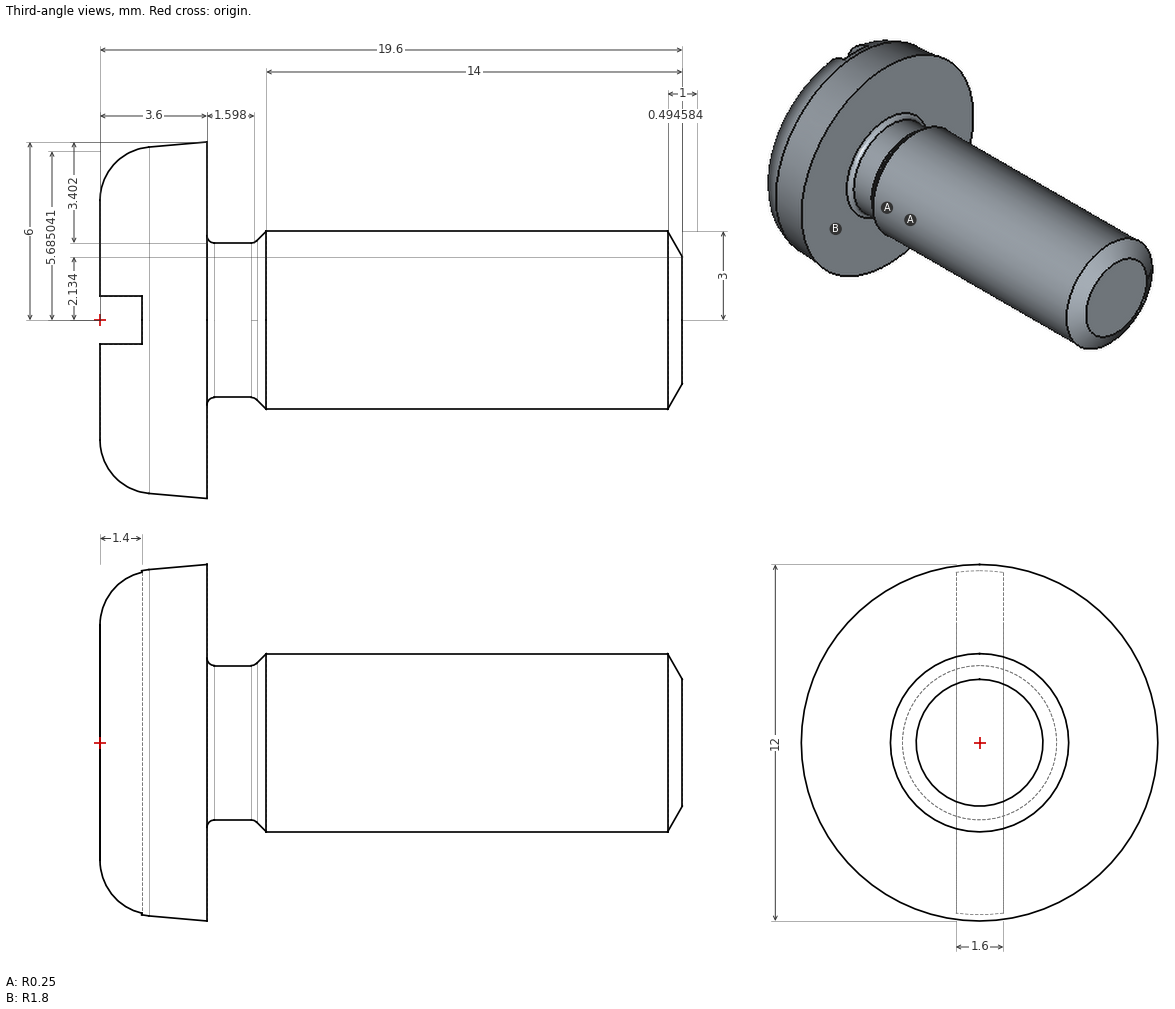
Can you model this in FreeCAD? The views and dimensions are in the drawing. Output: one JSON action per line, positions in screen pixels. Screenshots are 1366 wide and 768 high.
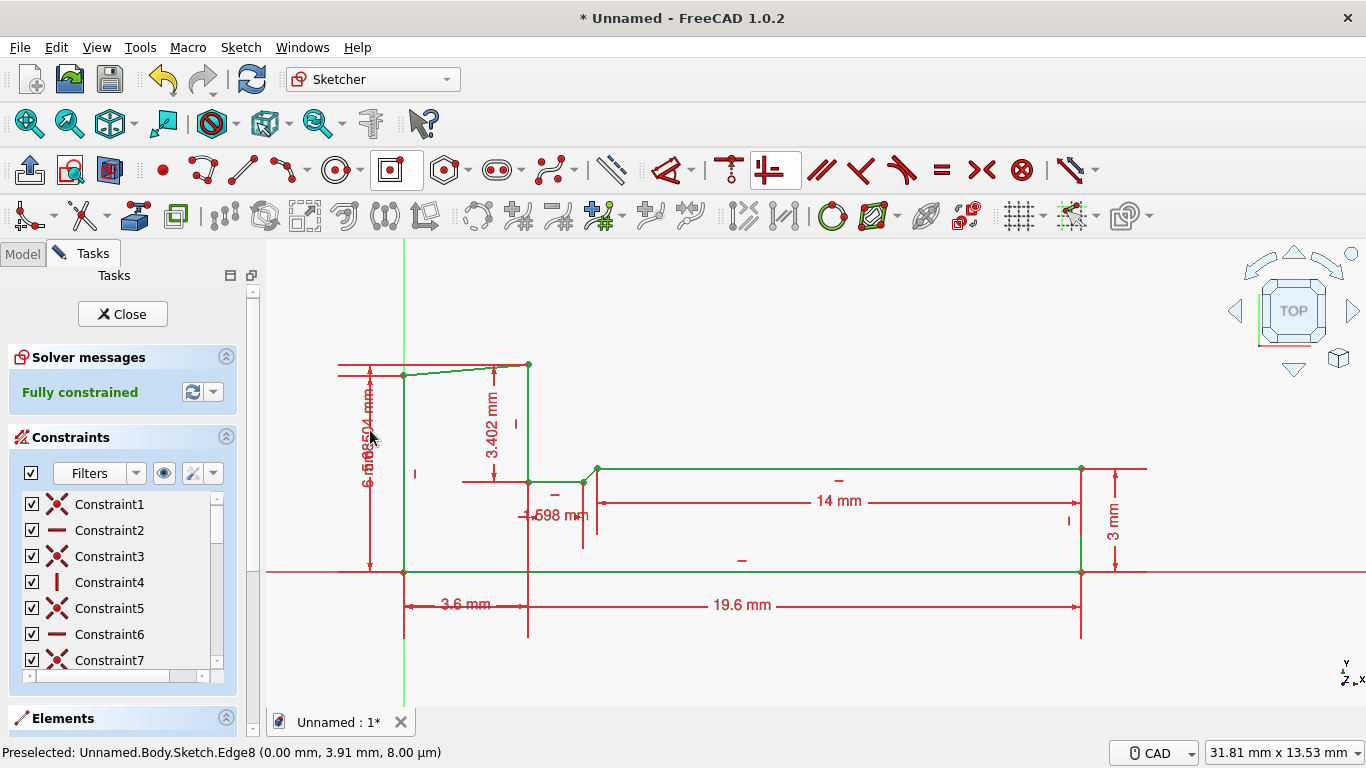
{"action": "left_click", "coordinate": [123, 314]}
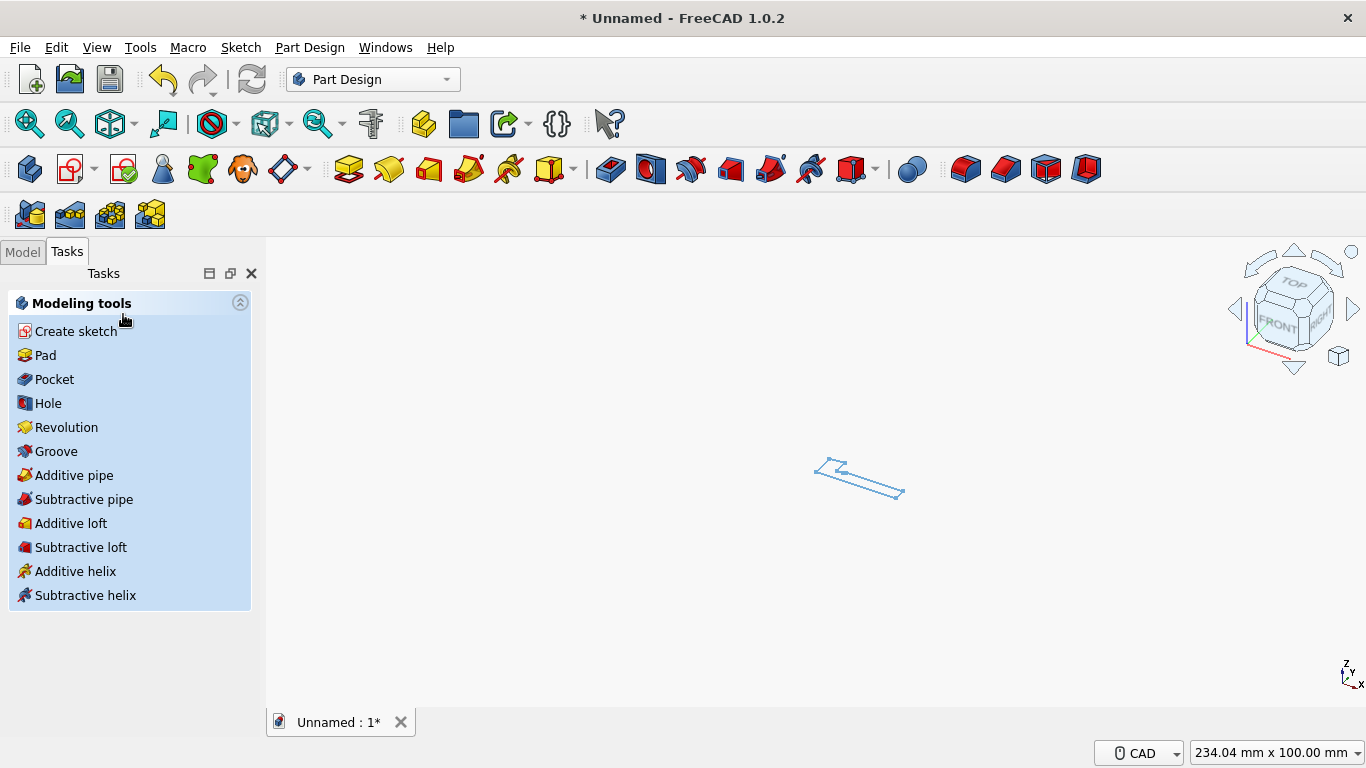
{"action": "left_click", "coordinate": [390, 170]}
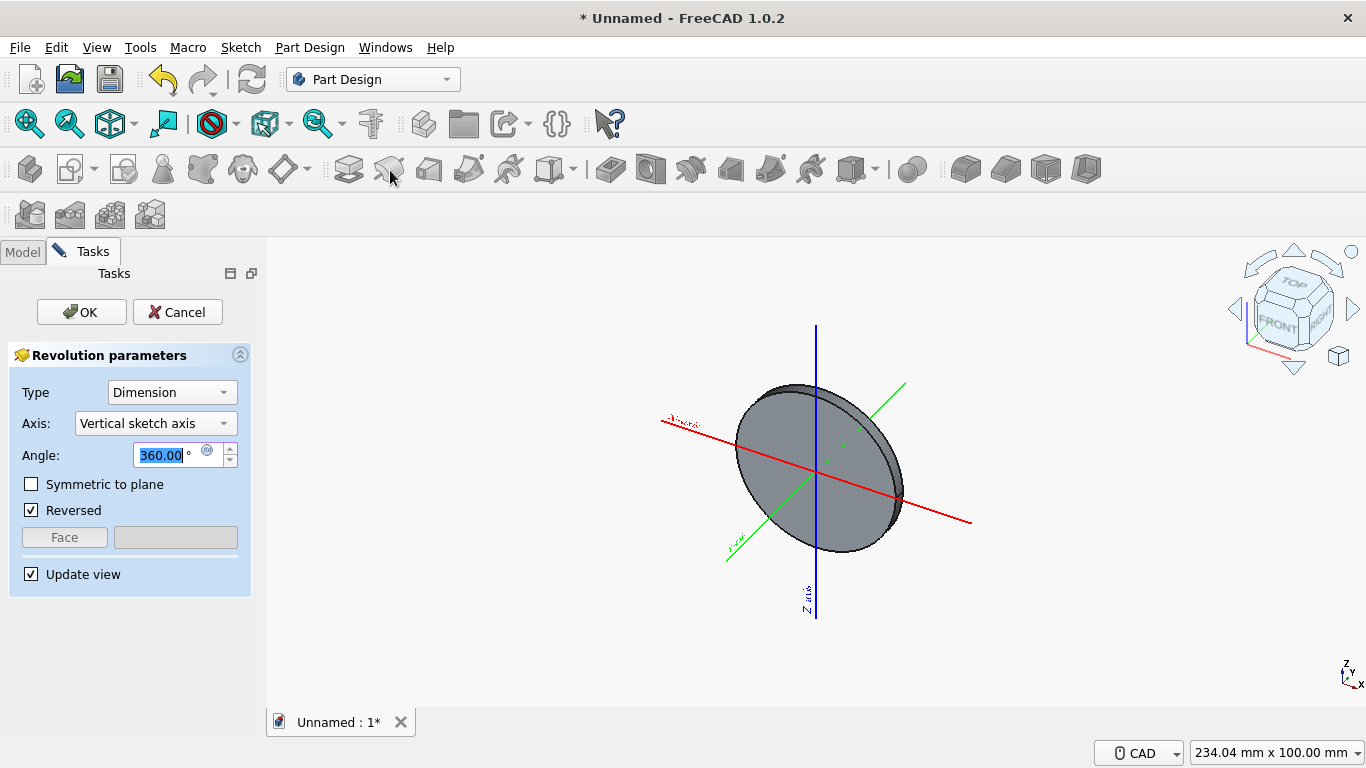
{"action": "left_click", "coordinate": [156, 424]}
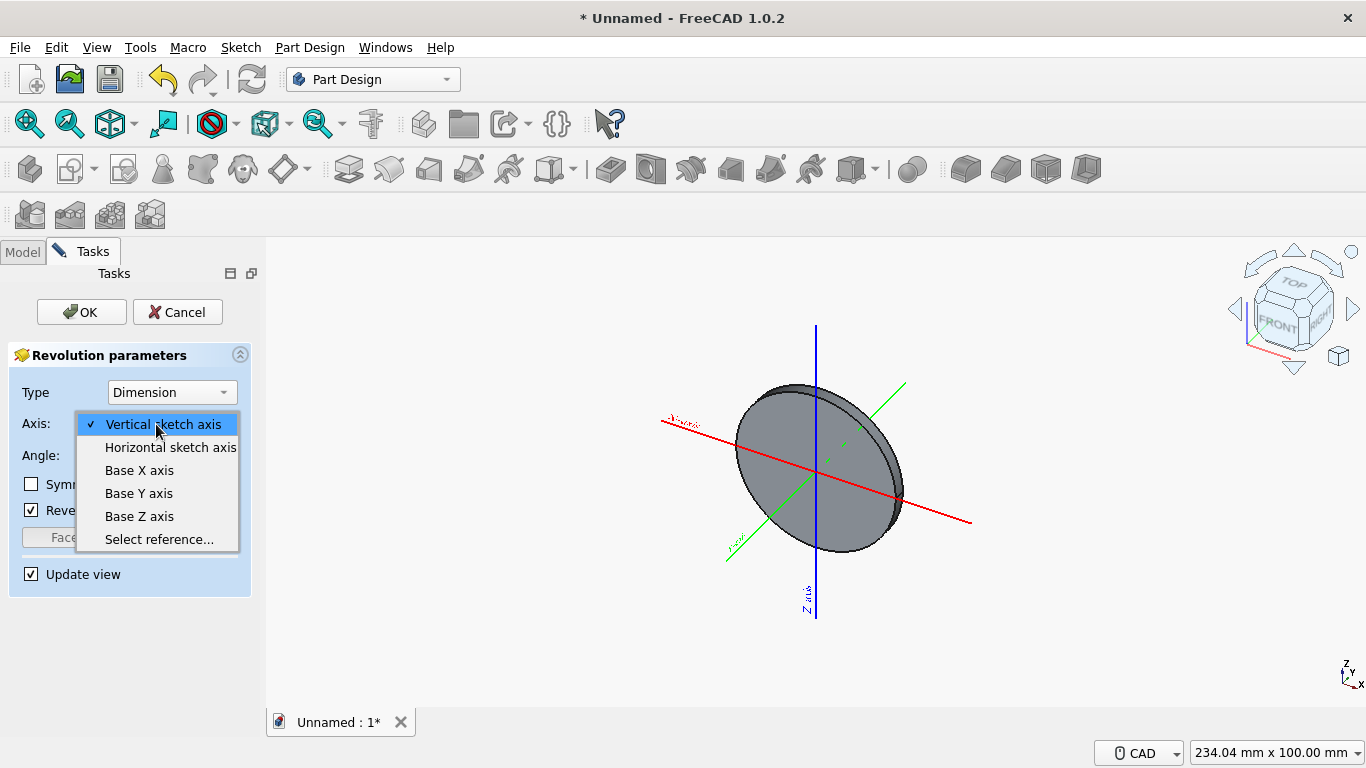
{"action": "left_click", "coordinate": [156, 448]}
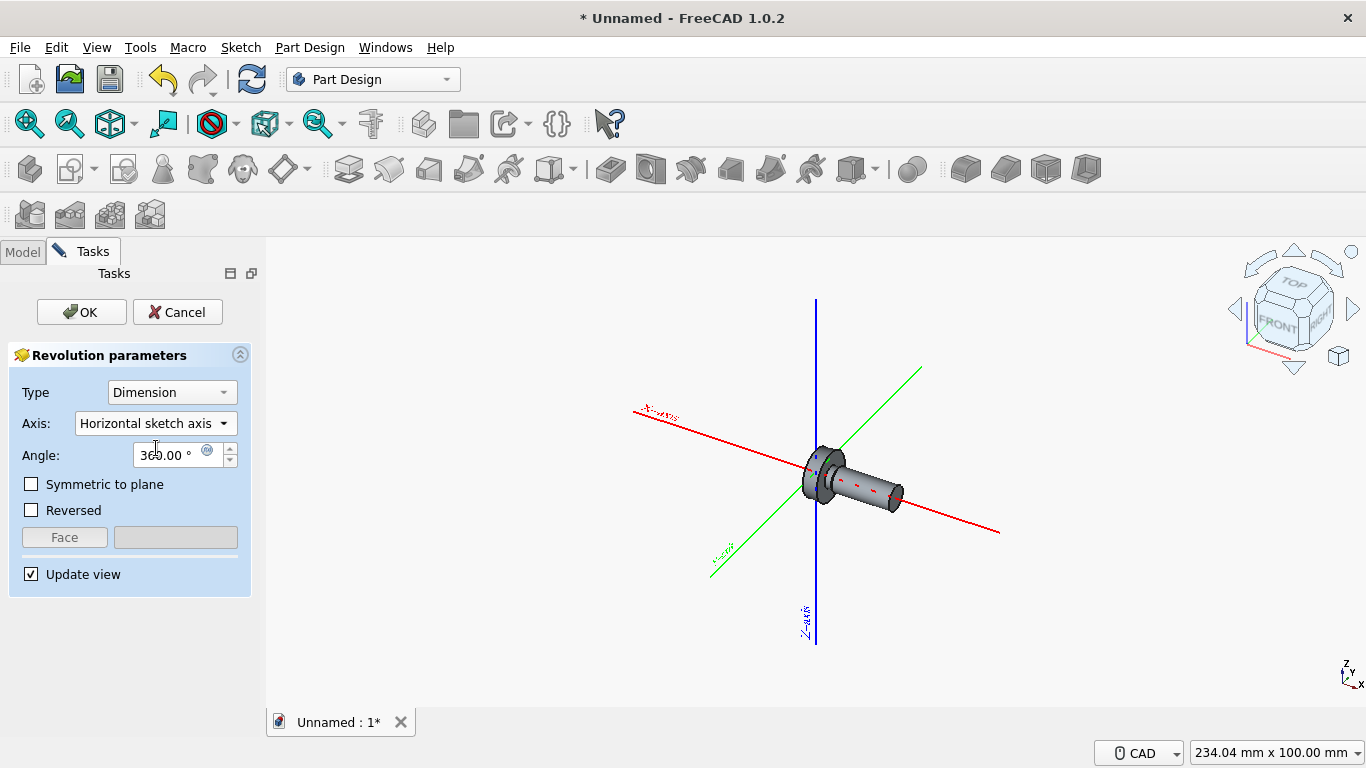
{"action": "left_click", "coordinate": [82, 312]}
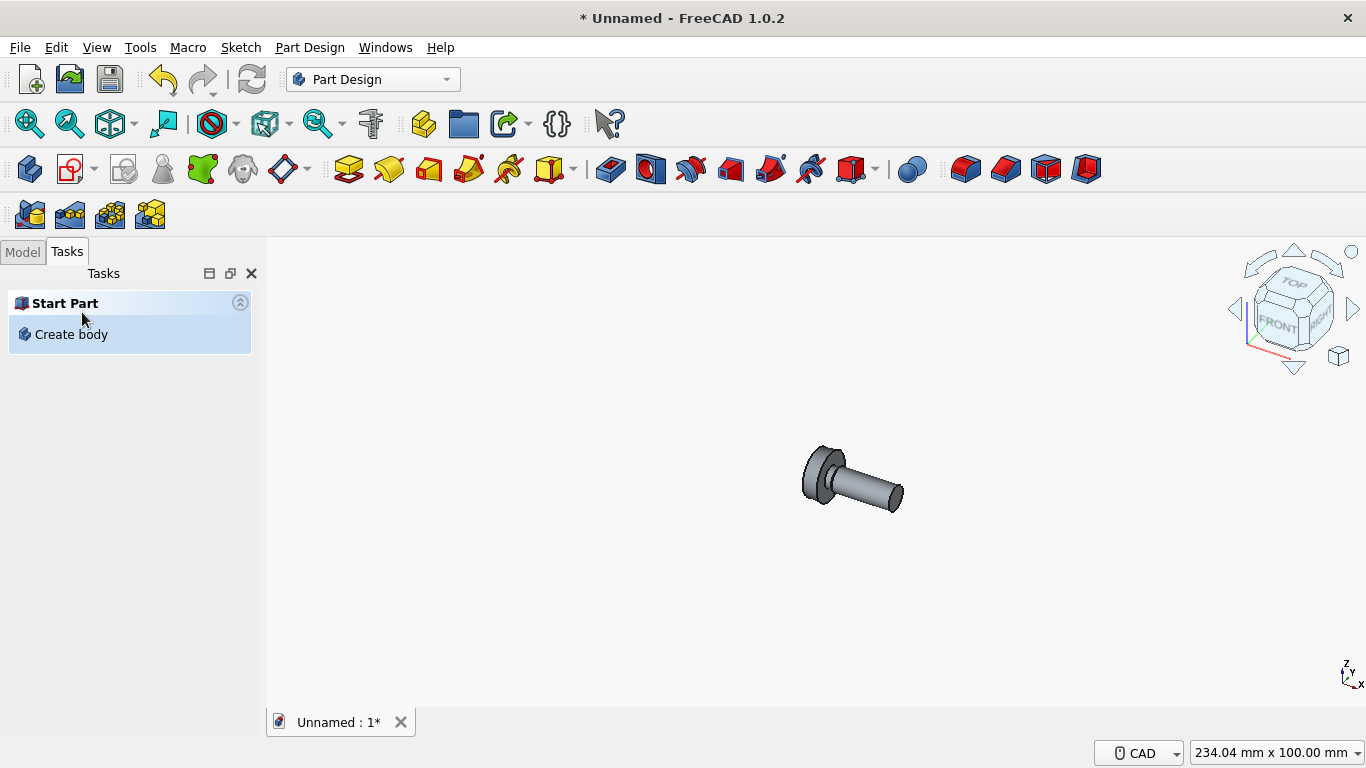
{"action": "left_click", "coordinate": [30, 124]}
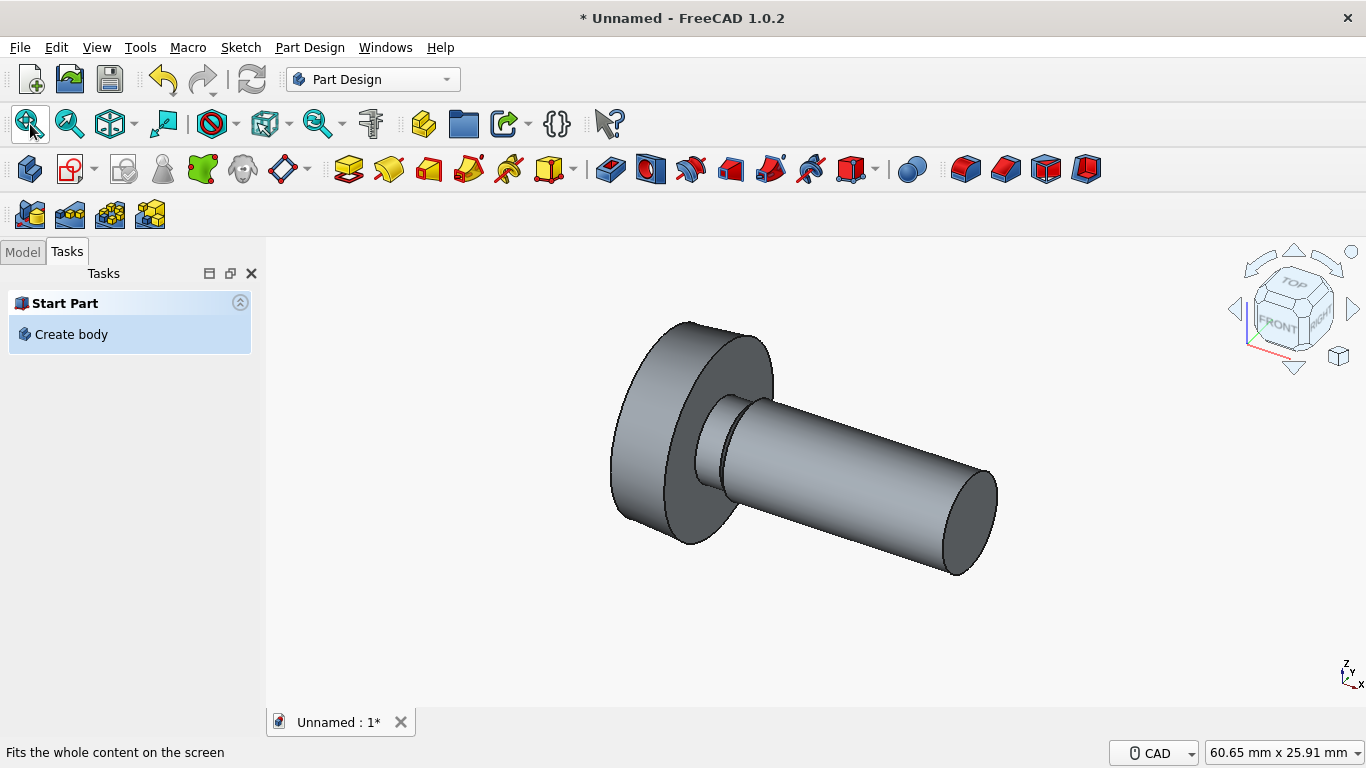
{"action": "key", "text": "0"}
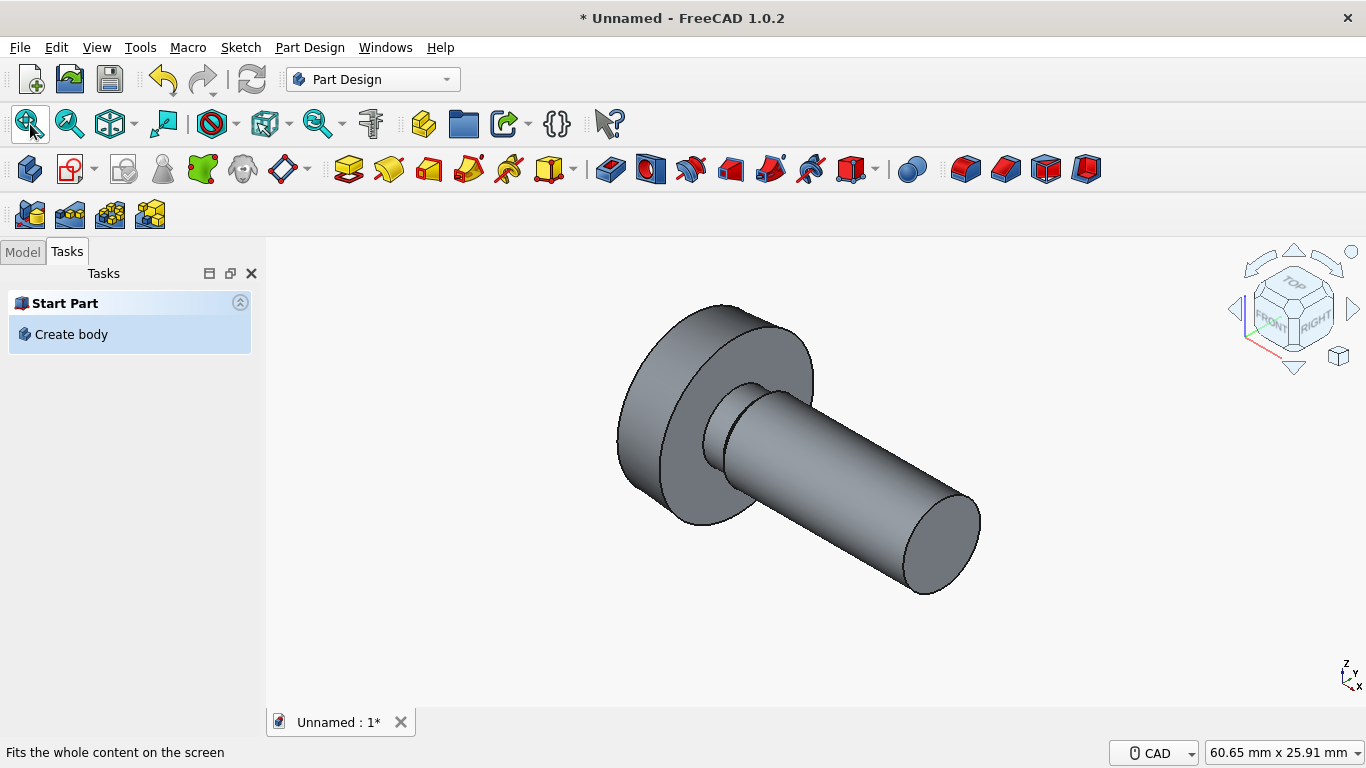
{"action": "key", "text": "2"}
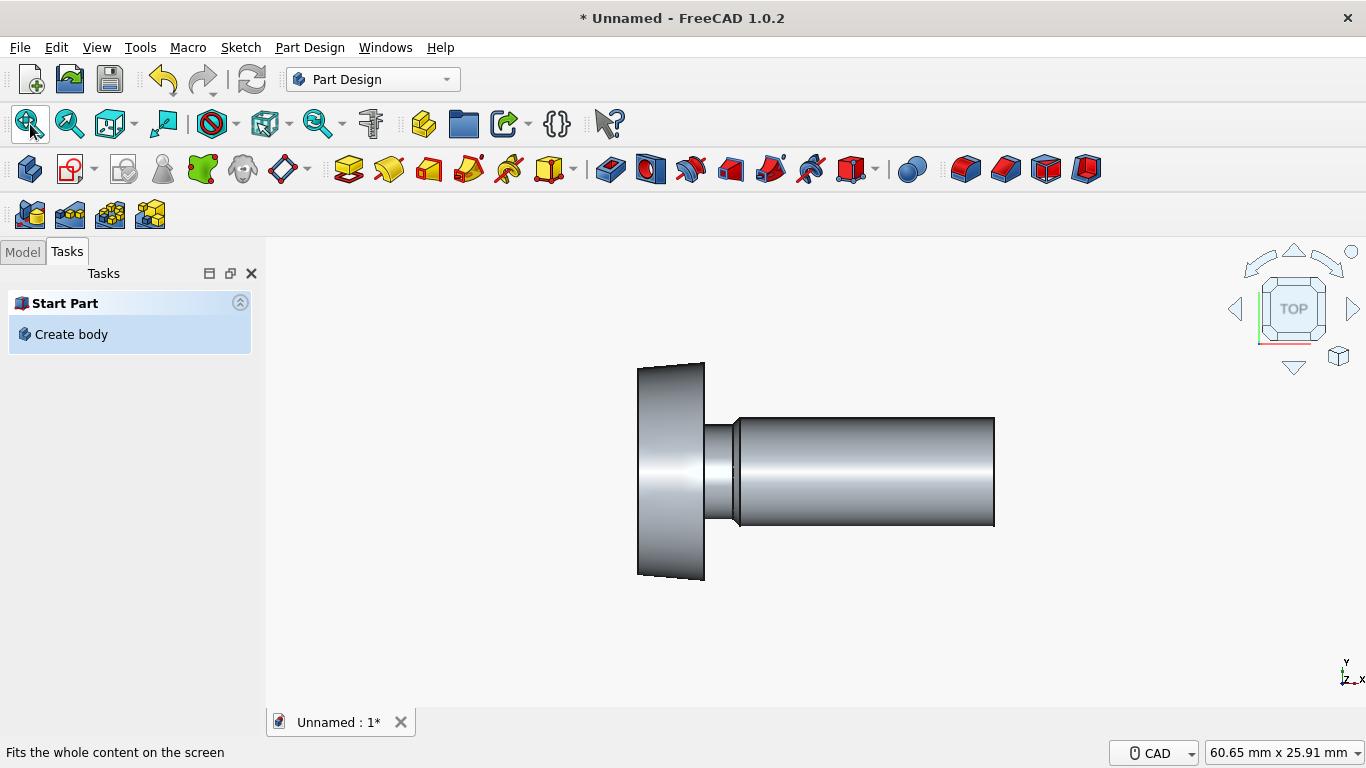
{"action": "key", "text": "1"}